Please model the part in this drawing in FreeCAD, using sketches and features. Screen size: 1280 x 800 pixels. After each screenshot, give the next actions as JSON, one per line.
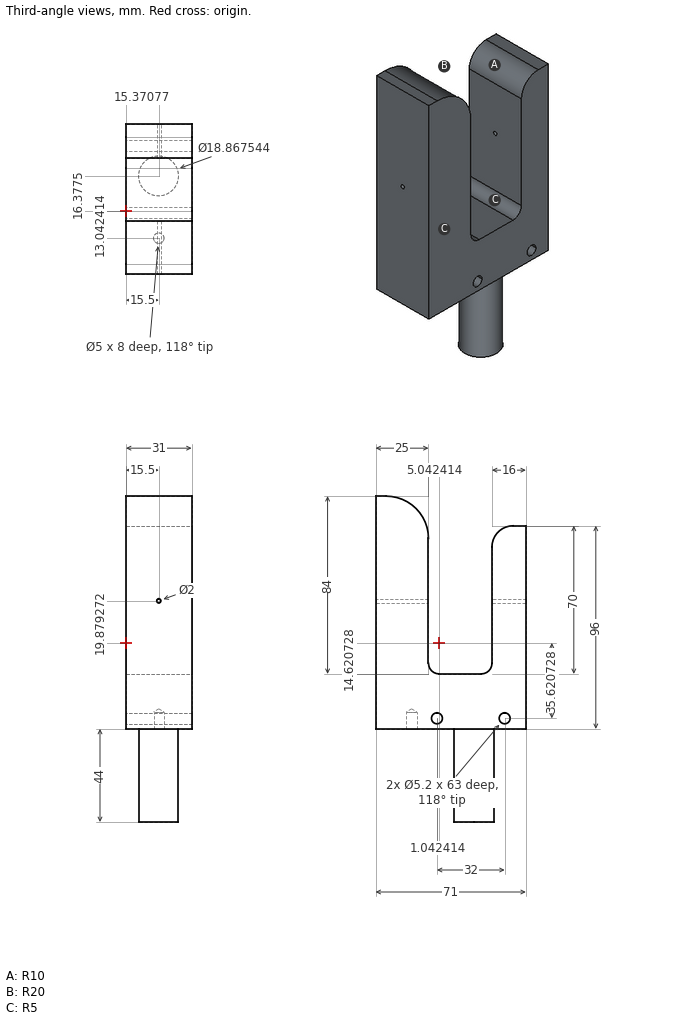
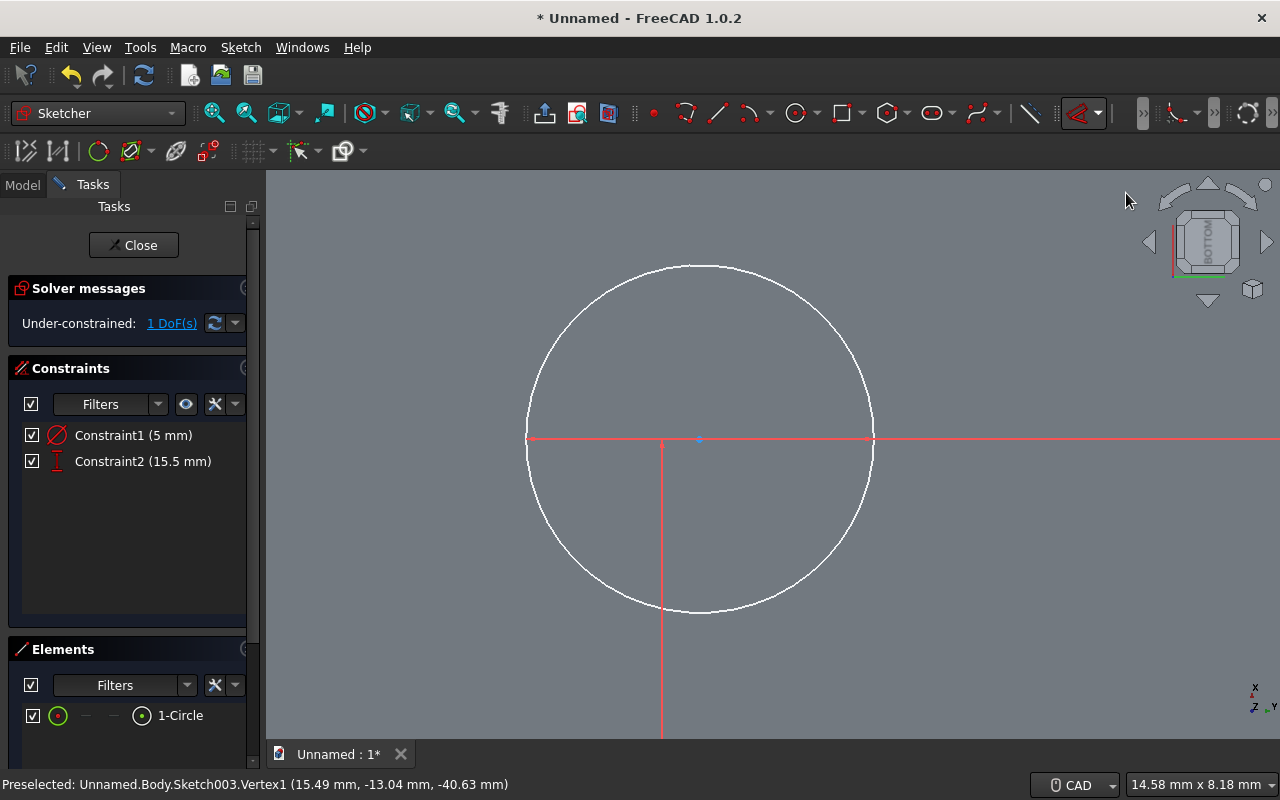
{"action": "left_click", "coordinate": [700, 439]}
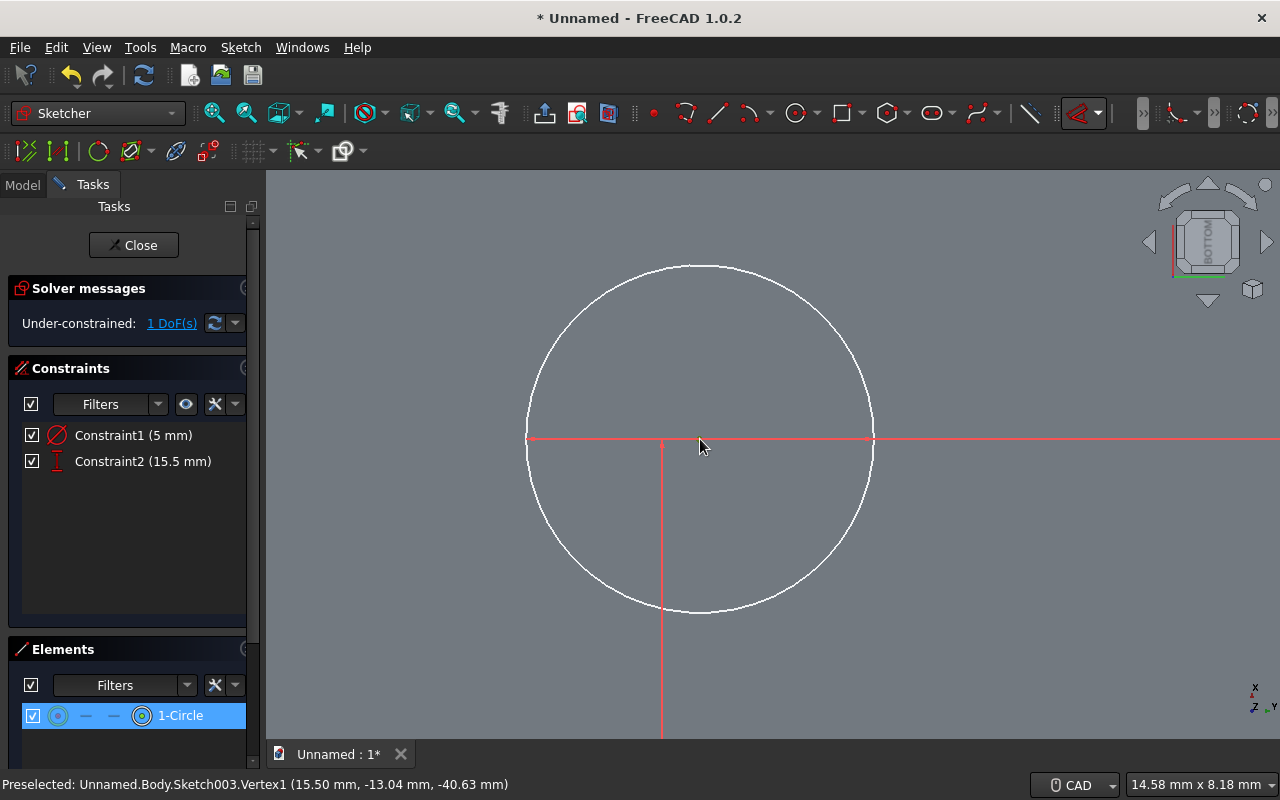
{"action": "left_click", "coordinate": [1100, 114]}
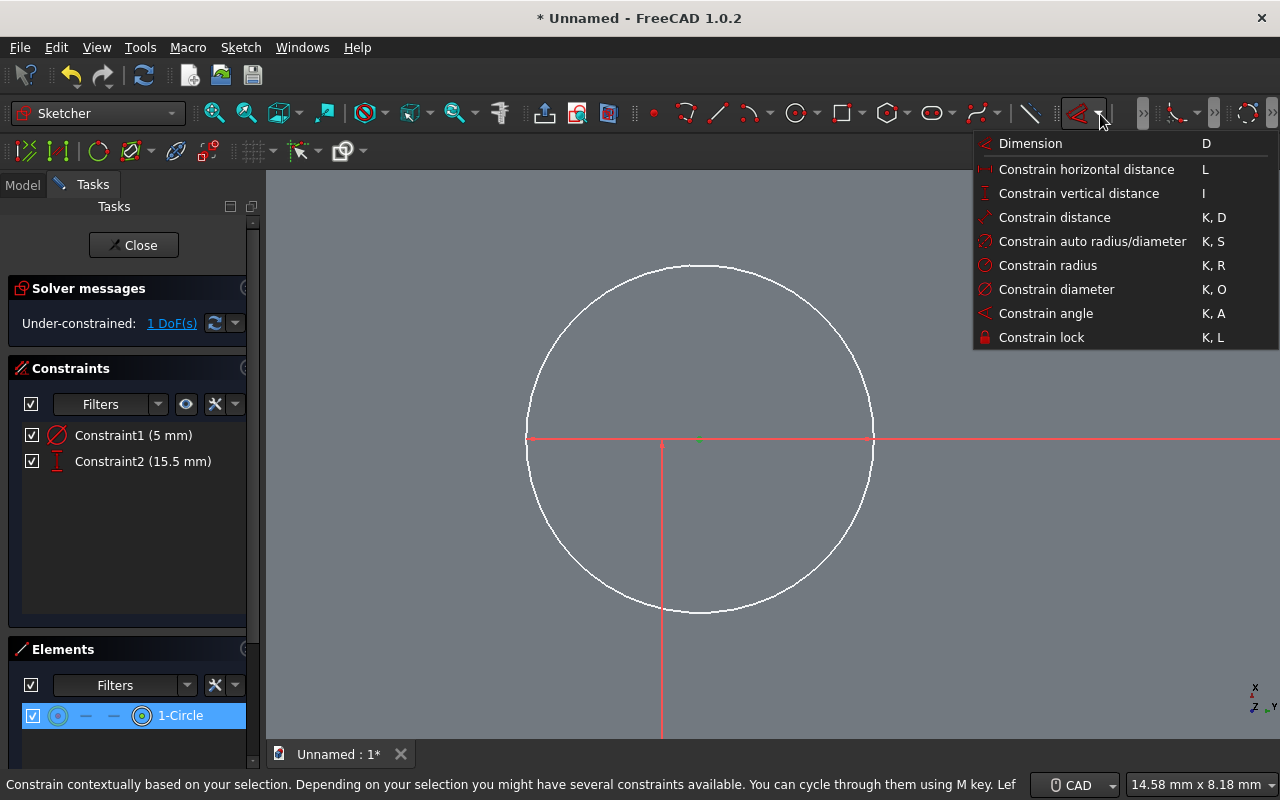
{"action": "left_click", "coordinate": [1126, 169]}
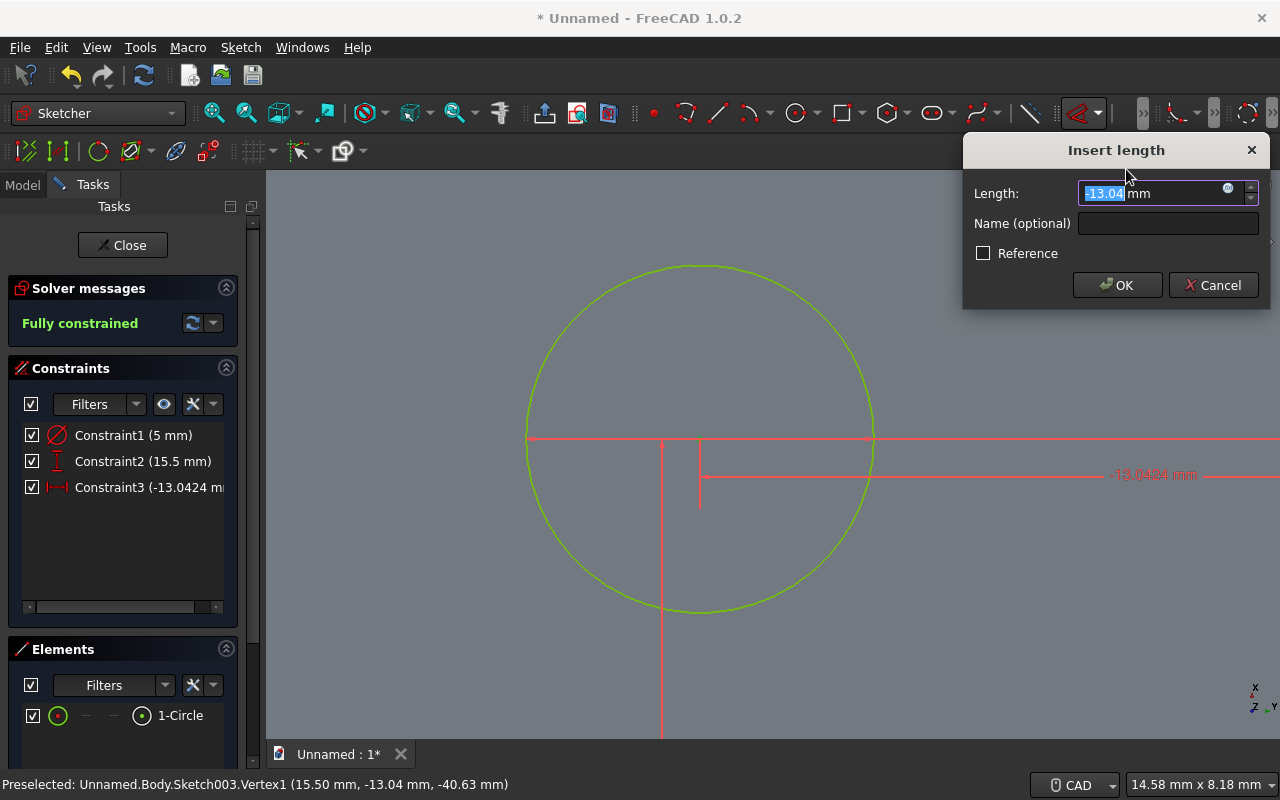
{"action": "type", "text": "-13.042414"}
{"action": "key", "text": "Return"}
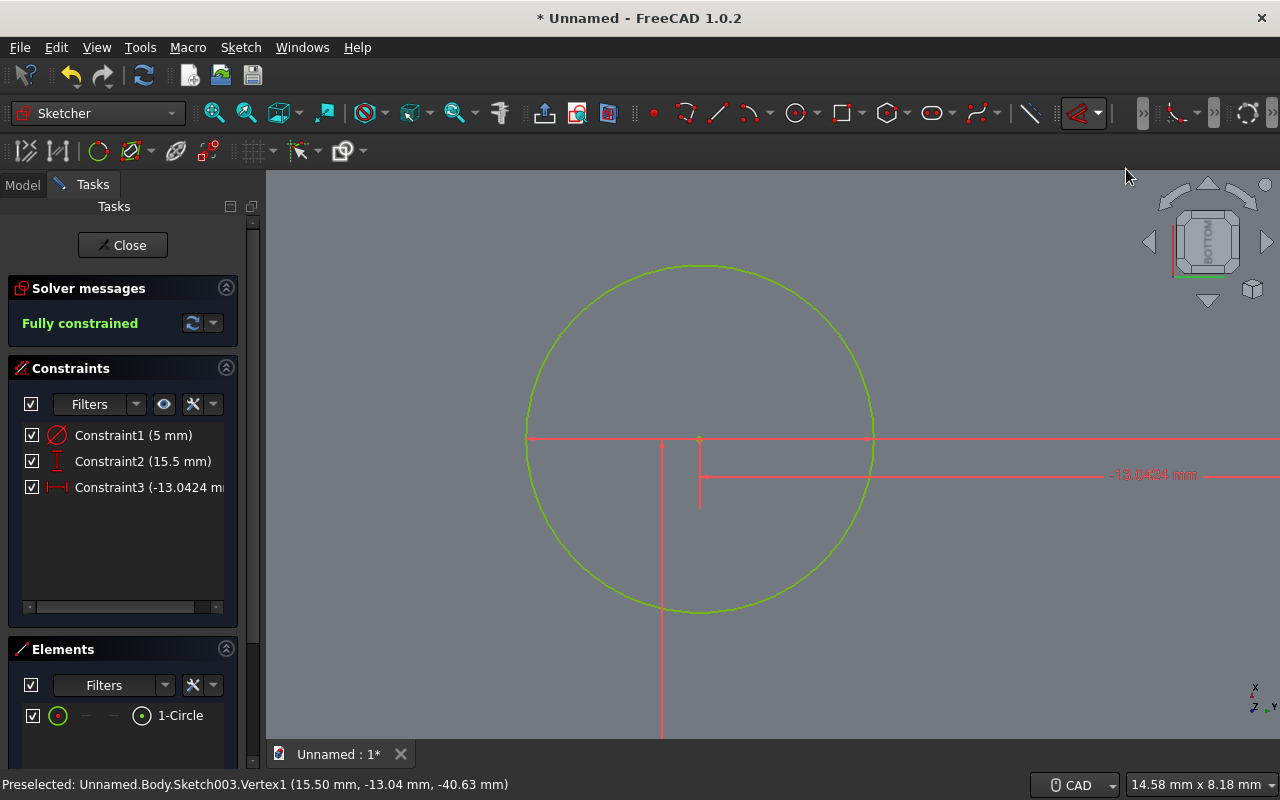
{"action": "left_click", "coordinate": [123, 245]}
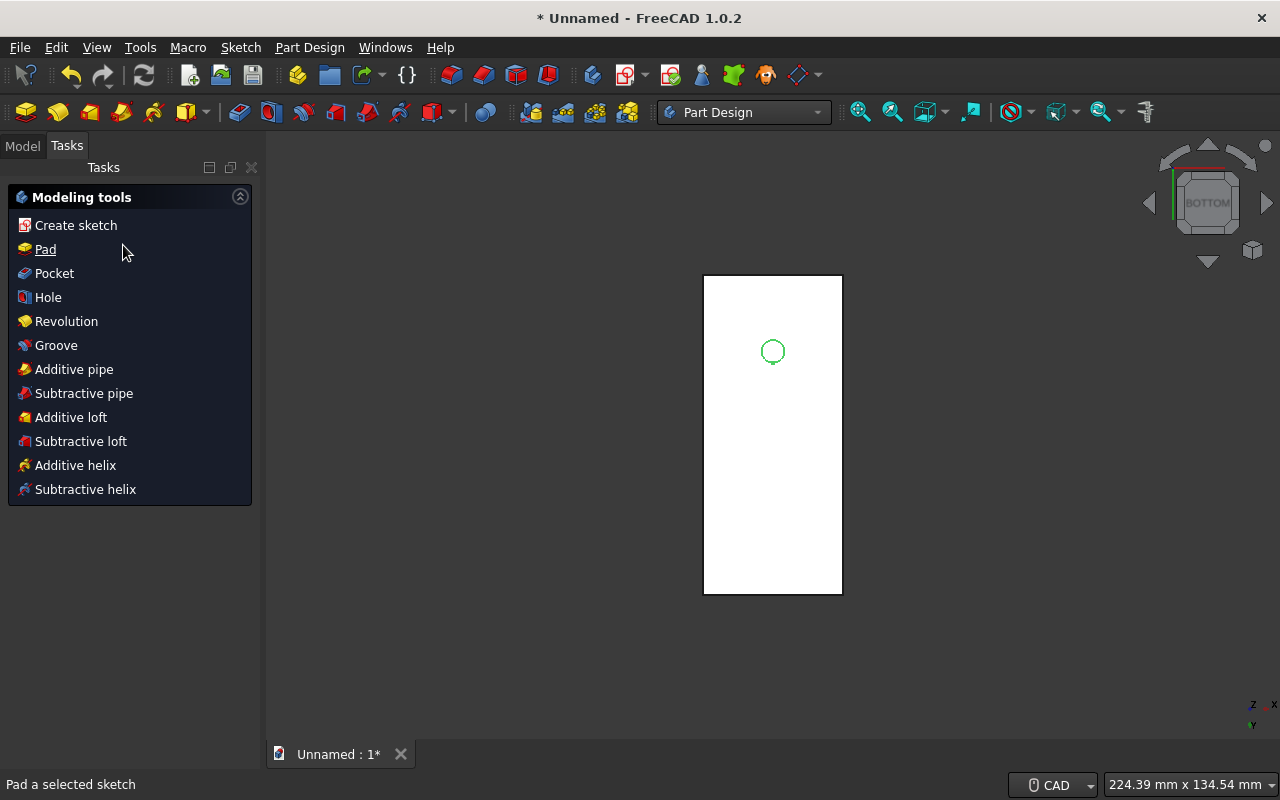
{"action": "left_click", "coordinate": [272, 112]}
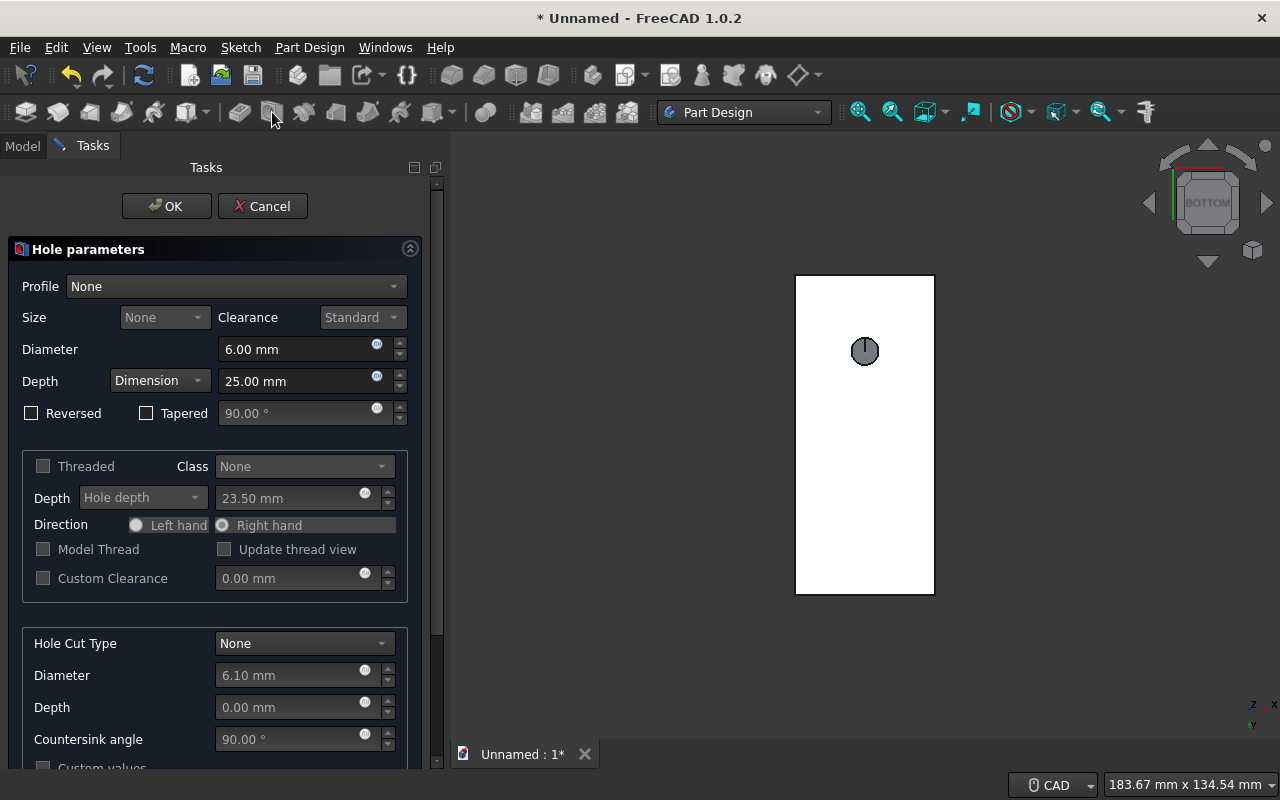
{"action": "triple_click", "coordinate": [305, 349]}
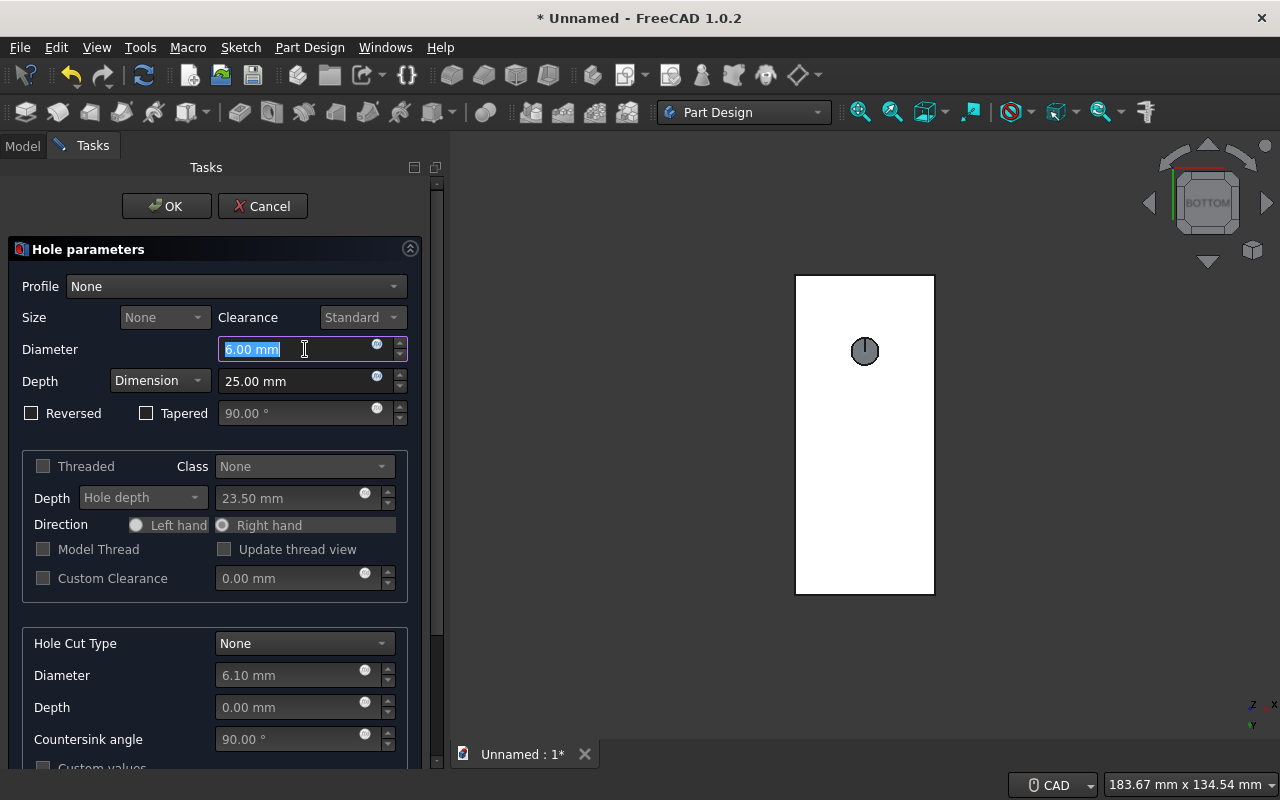
{"action": "type", "text": "5"}
{"action": "key", "text": "Tab"}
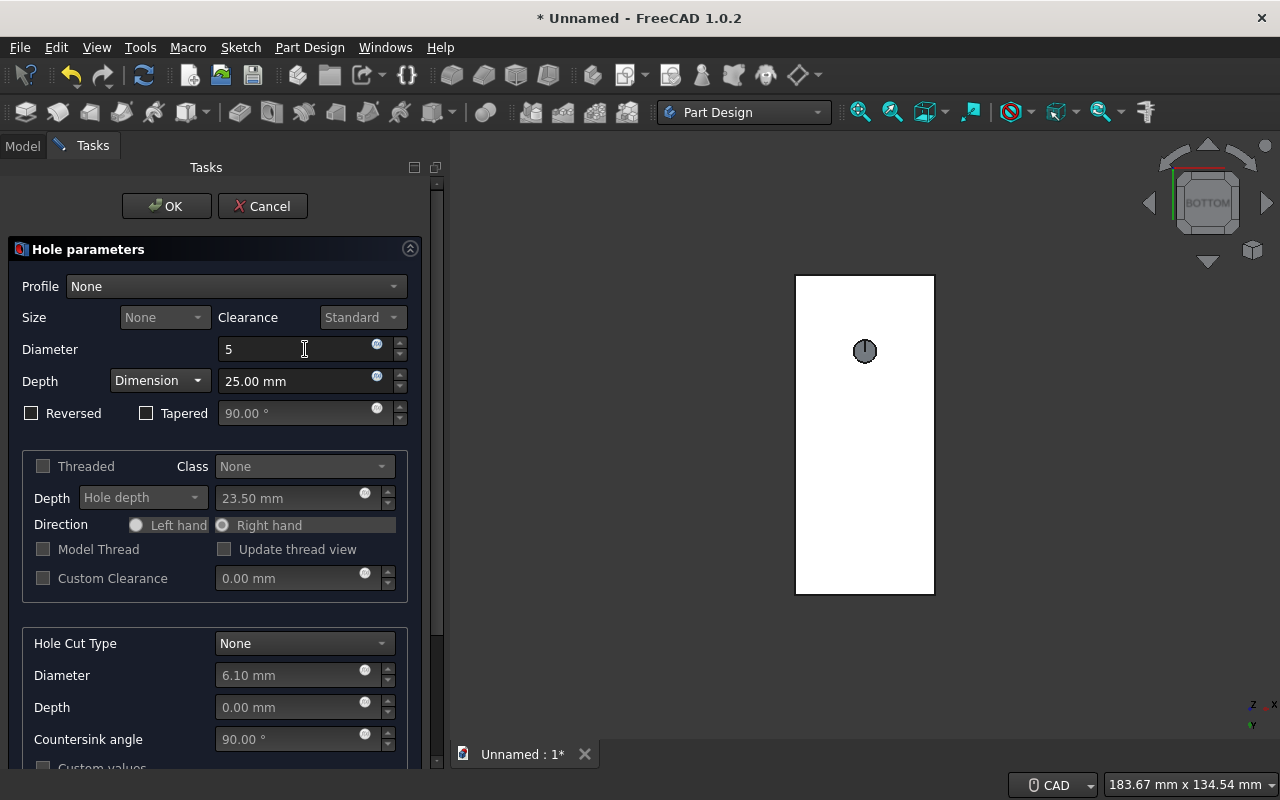
{"action": "triple_click", "coordinate": [305, 381]}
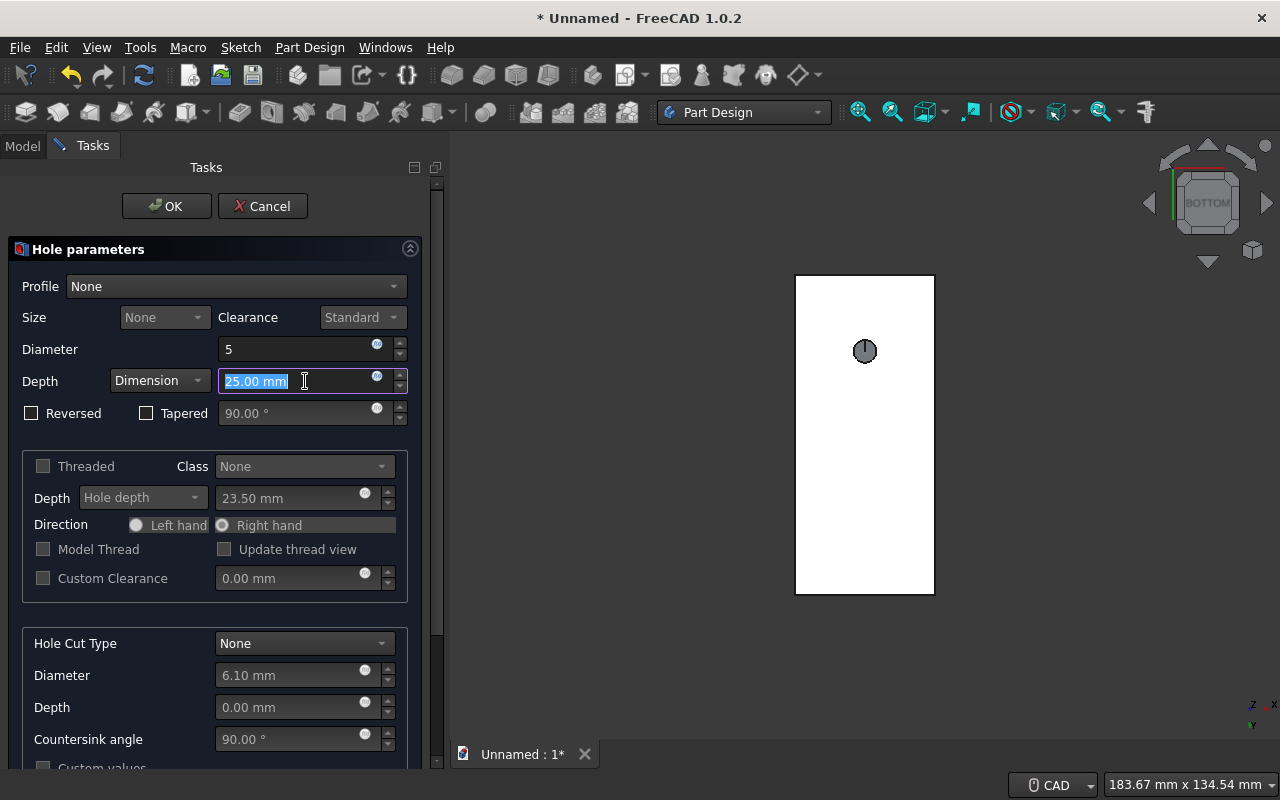
{"action": "type", "text": "8"}
{"action": "key", "text": "Tab"}